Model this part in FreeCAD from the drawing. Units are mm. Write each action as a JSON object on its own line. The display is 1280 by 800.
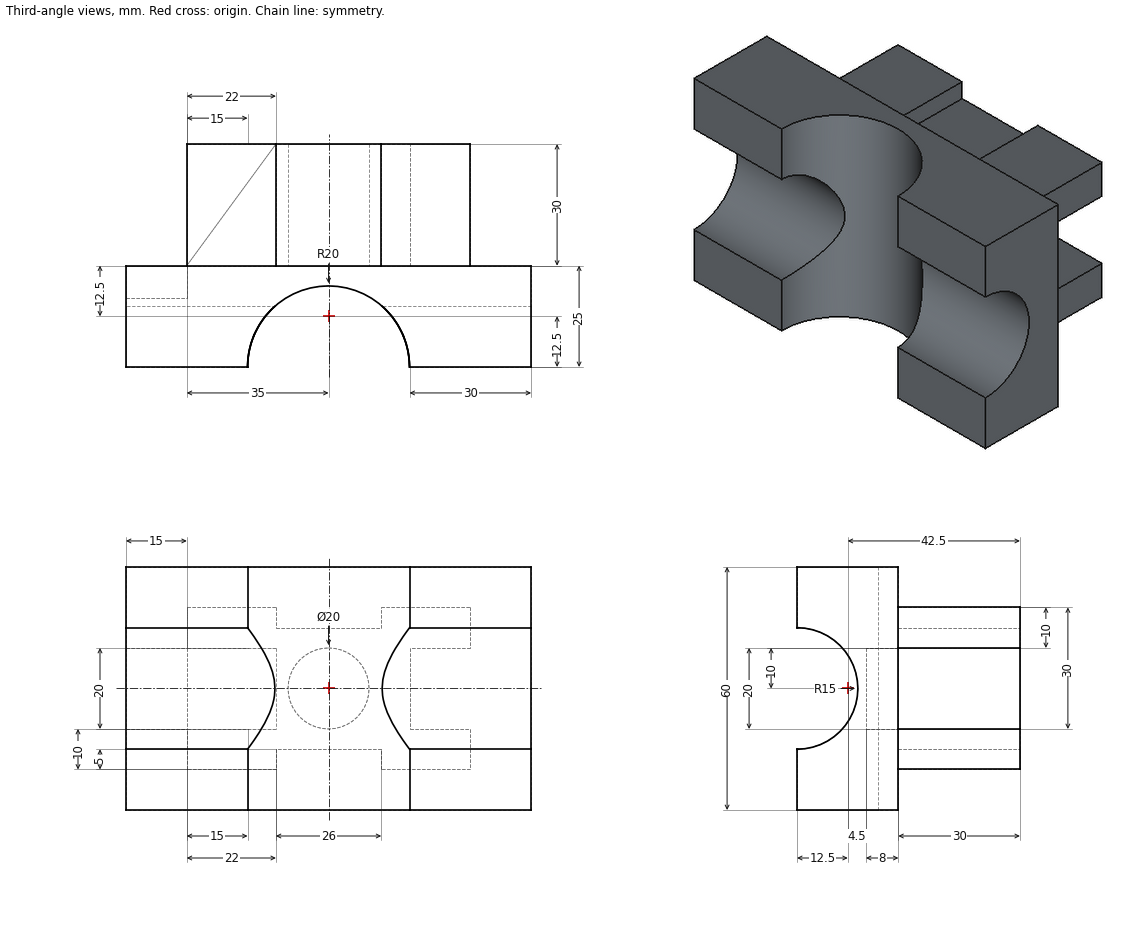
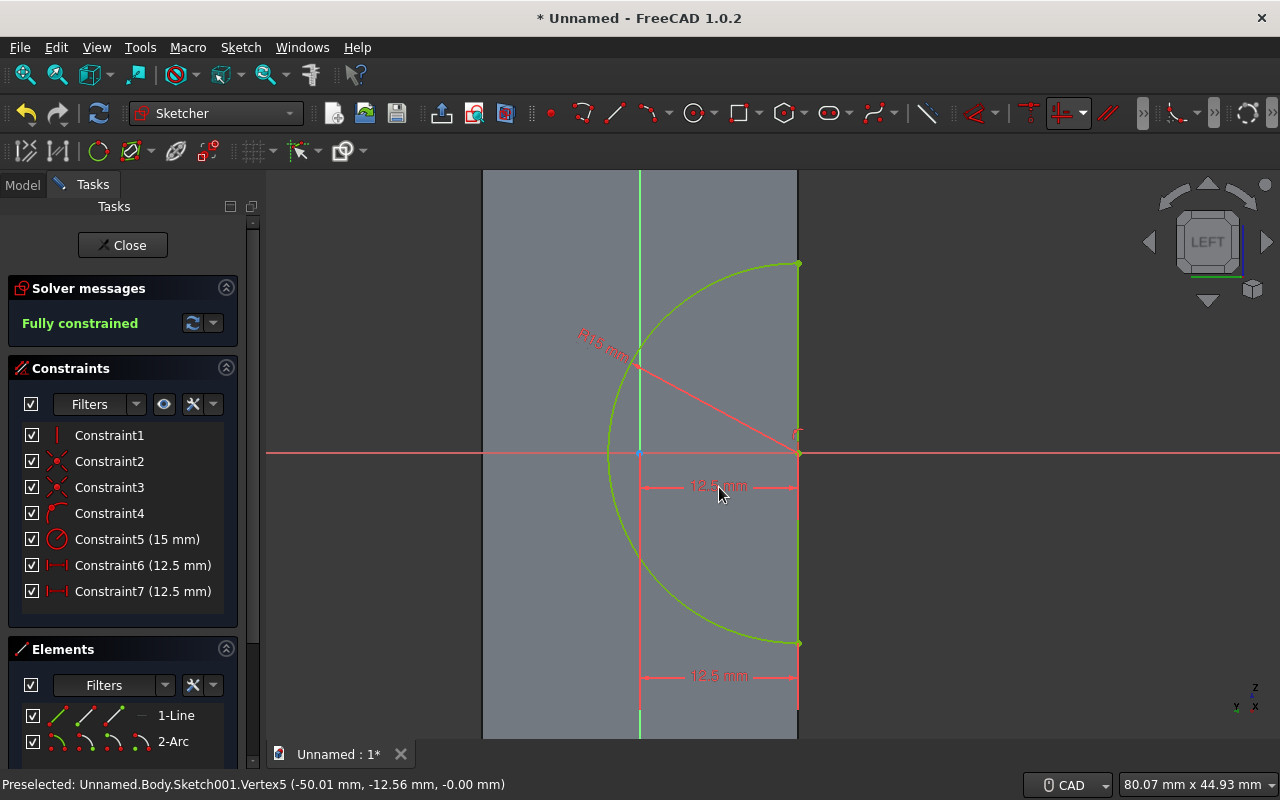
{"action": "left_click", "coordinate": [123, 245]}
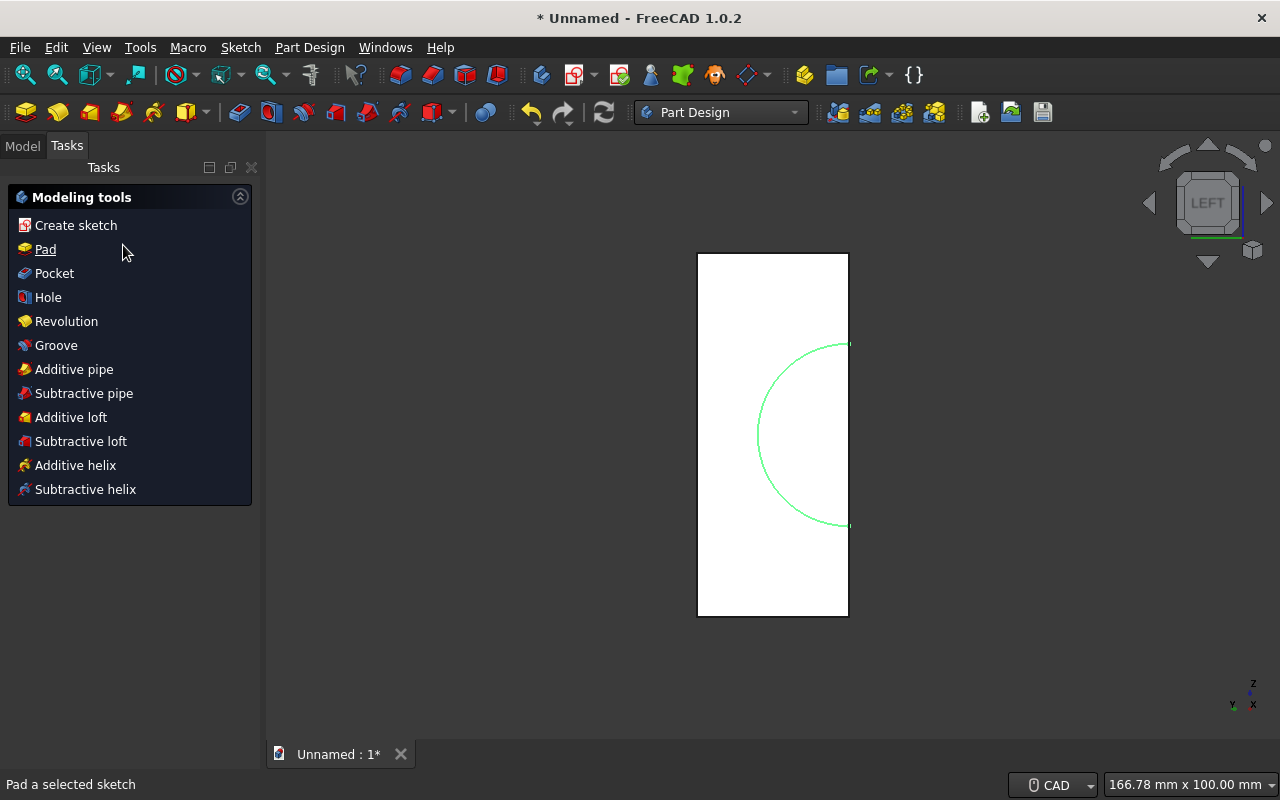
{"action": "left_click", "coordinate": [240, 112]}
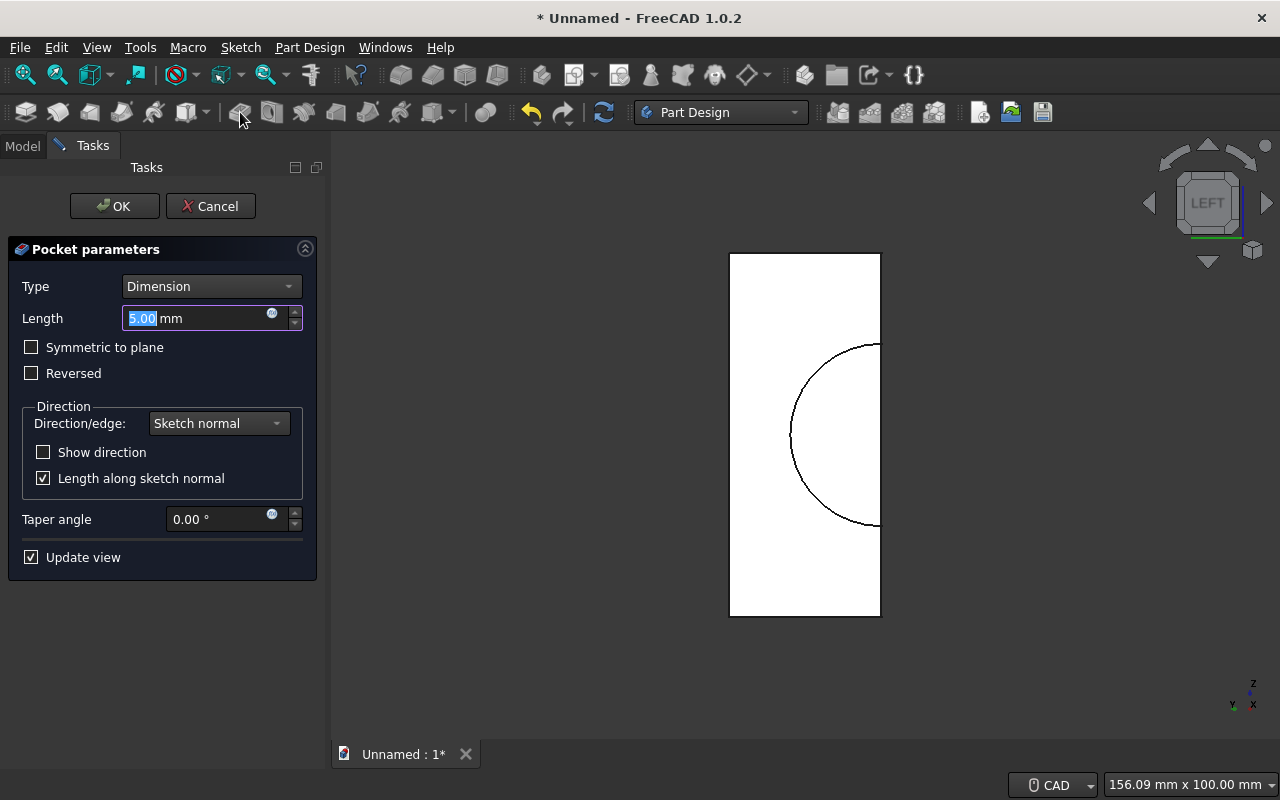
{"action": "left_click", "coordinate": [212, 286]}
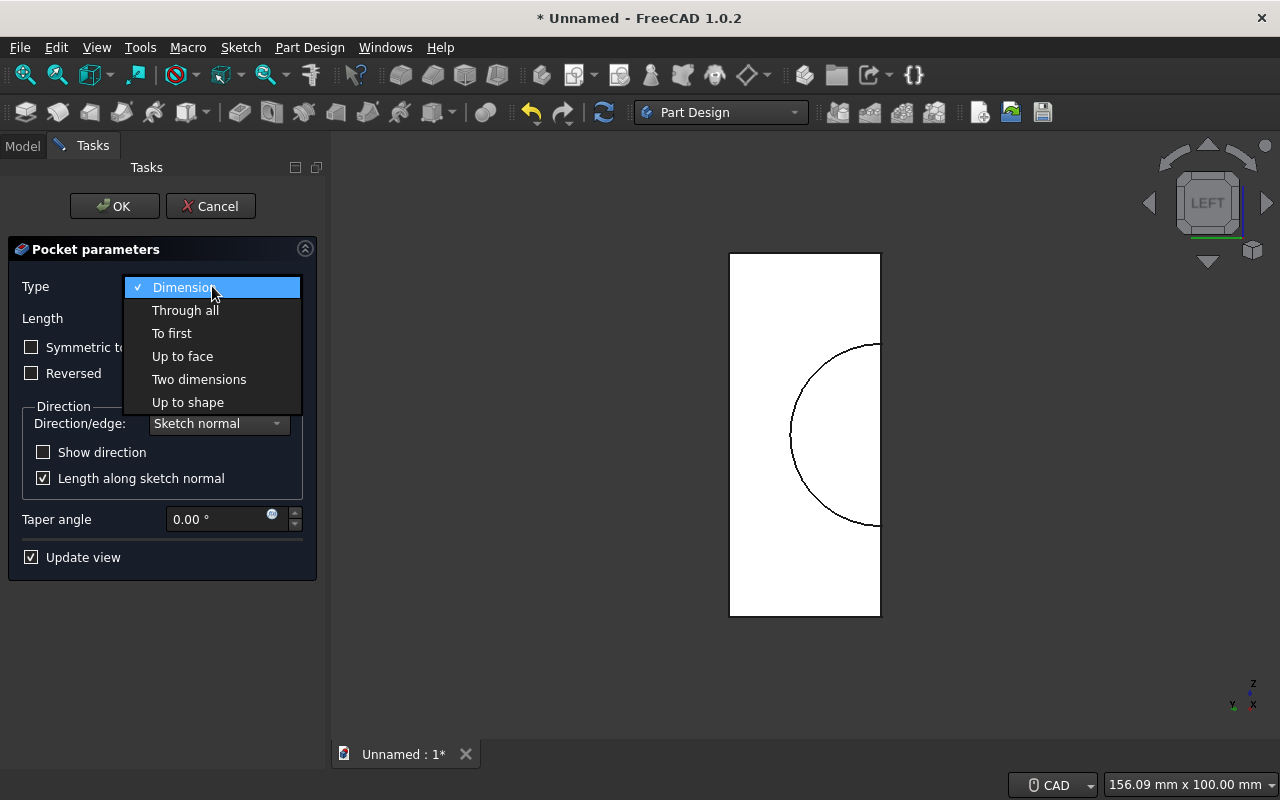
{"action": "left_click", "coordinate": [212, 310]}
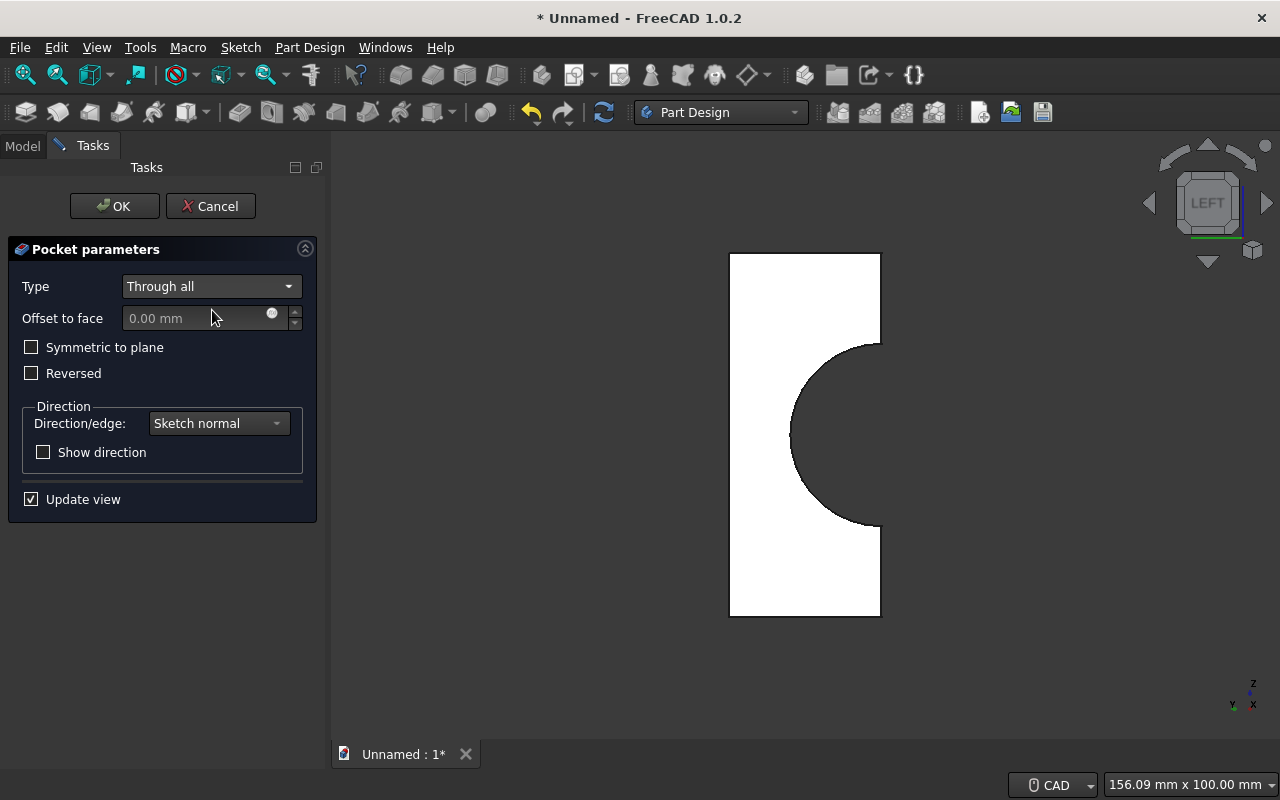
{"action": "left_click", "coordinate": [115, 206]}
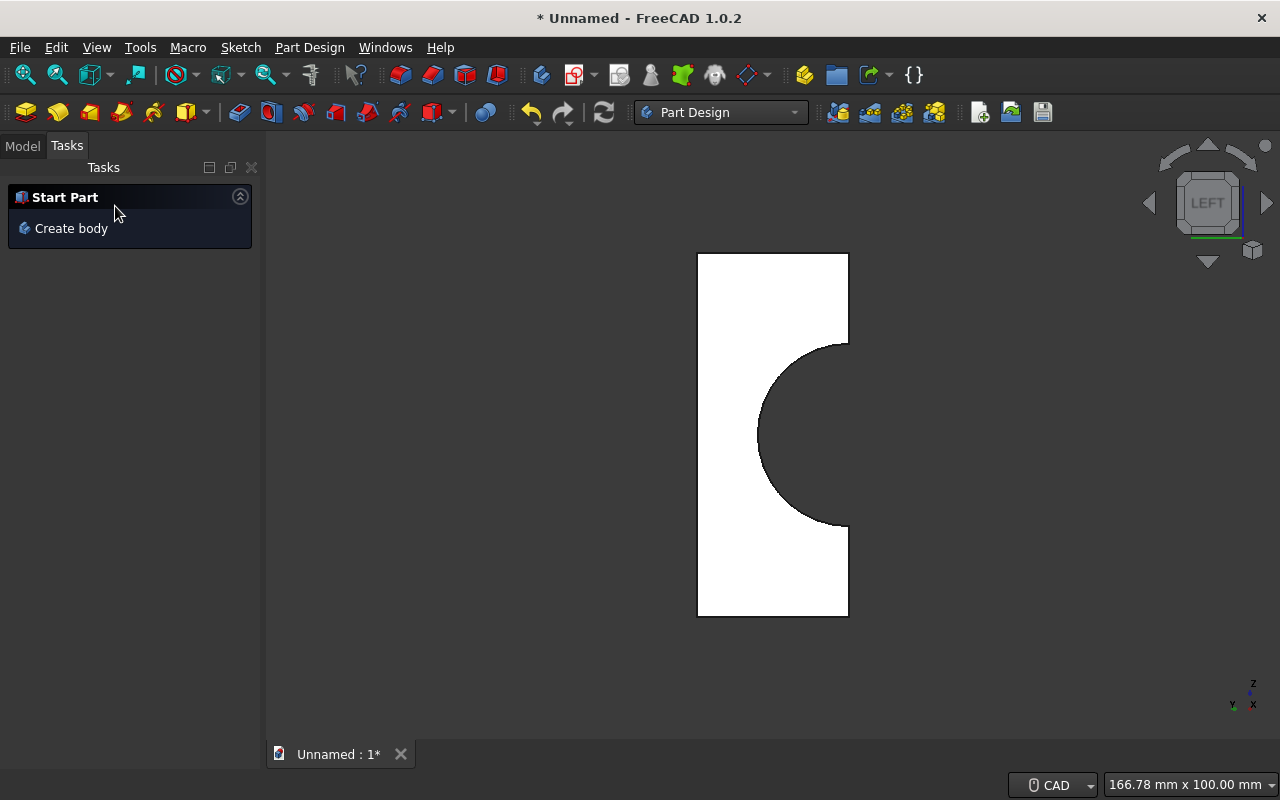
{"action": "left_click", "coordinate": [751, 538]}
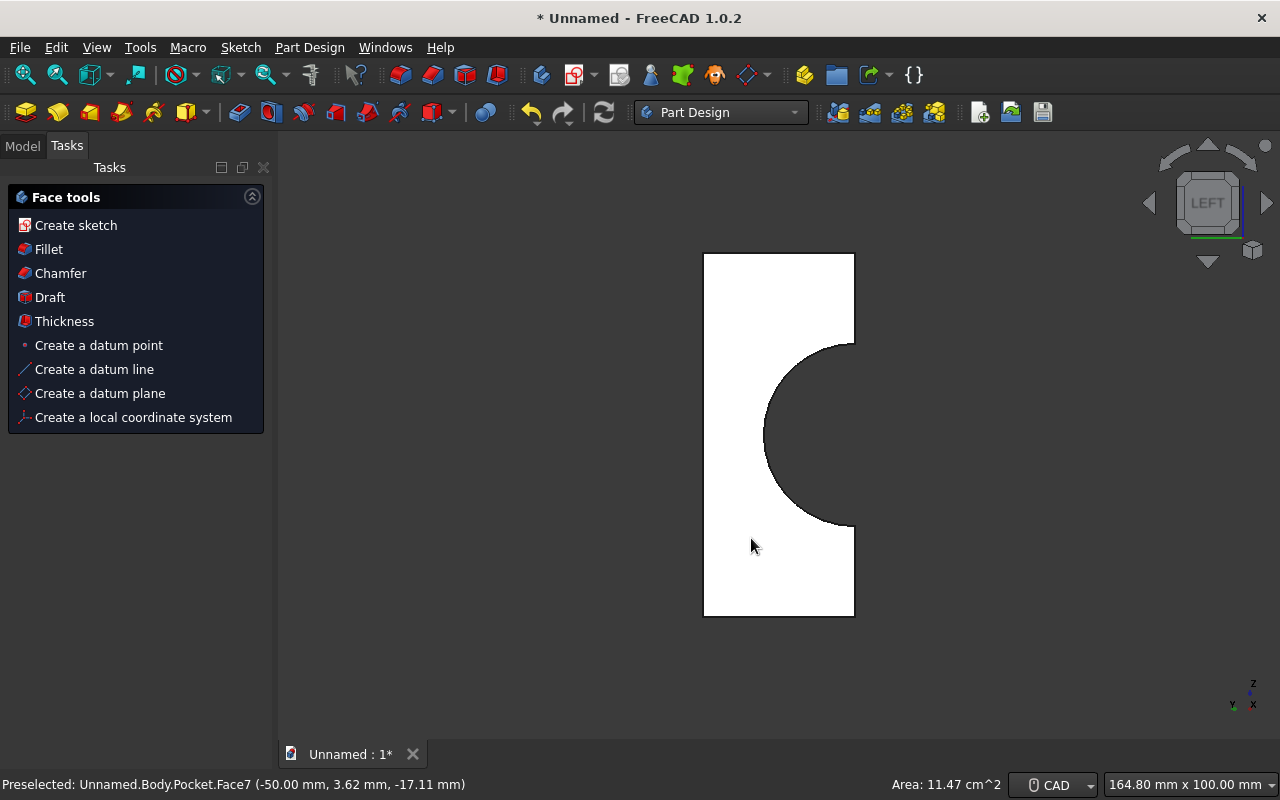
{"action": "left_click", "coordinate": [574, 76]}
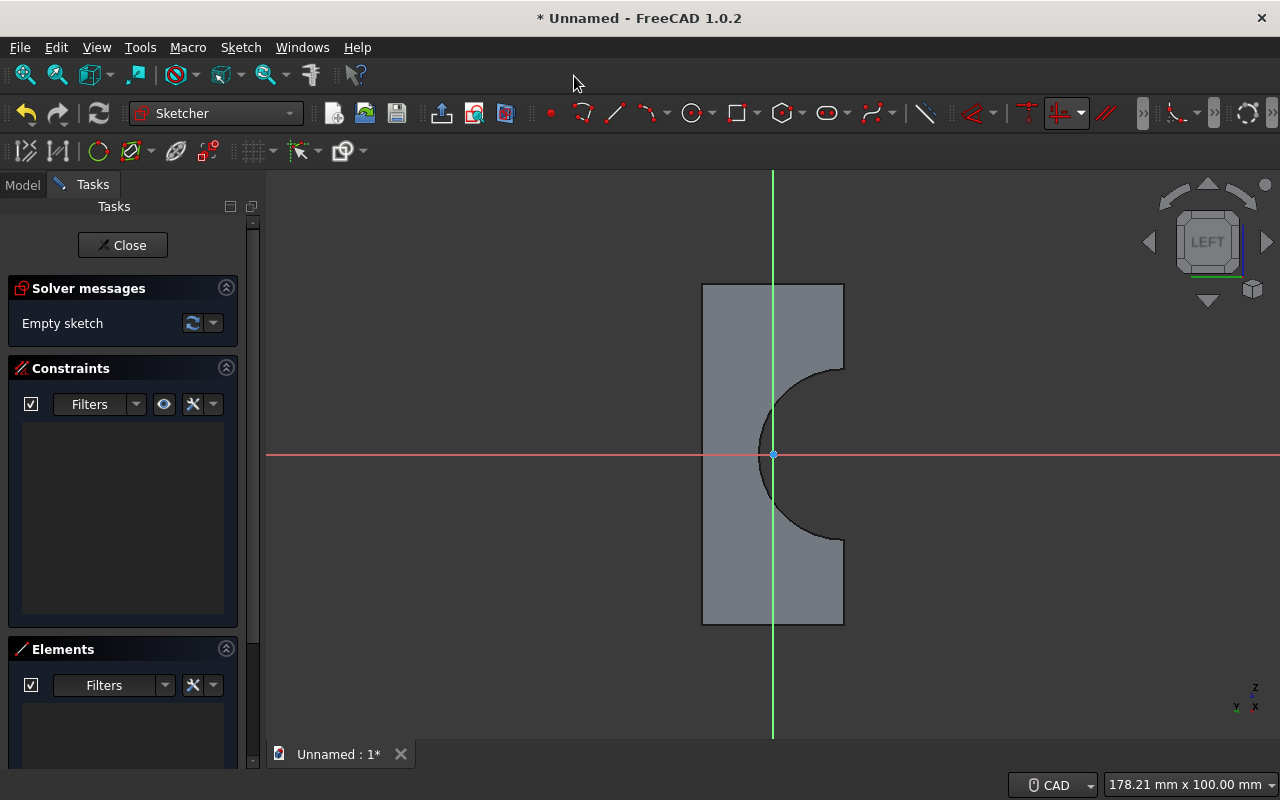
{"action": "scroll", "coordinate": [752, 455], "scroll_direction": "up", "scroll_amount": 6}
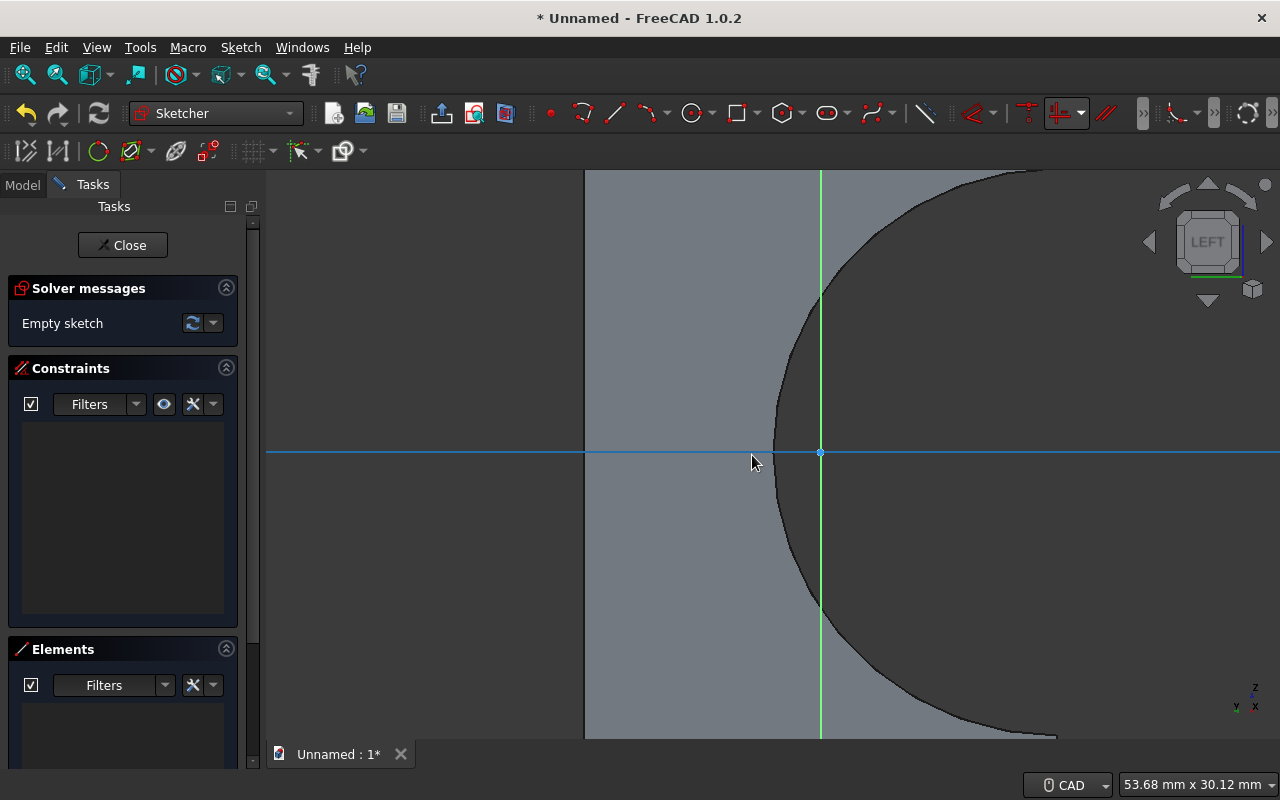
{"action": "left_click", "coordinate": [738, 114]}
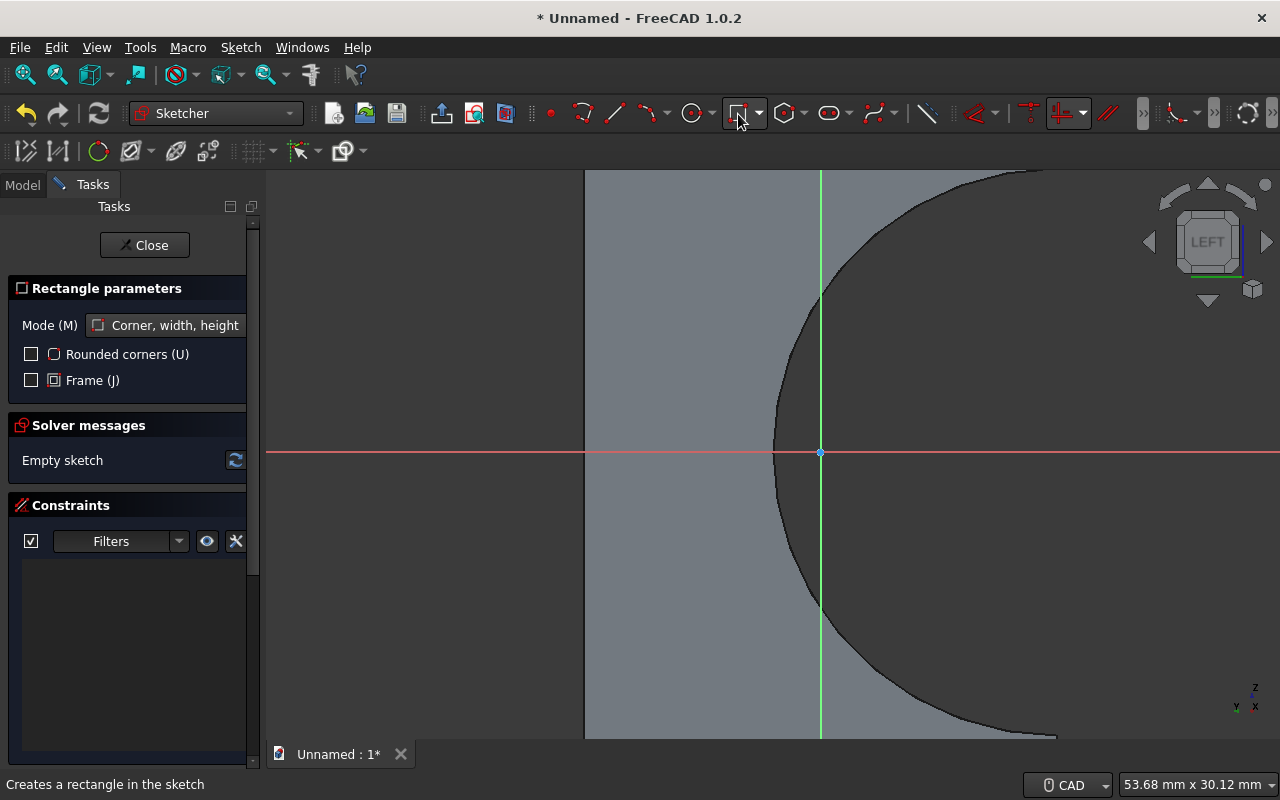
{"action": "left_click", "coordinate": [584, 263]}
{"action": "left_click", "coordinate": [736, 641]}
{"action": "key", "text": "Escape"}